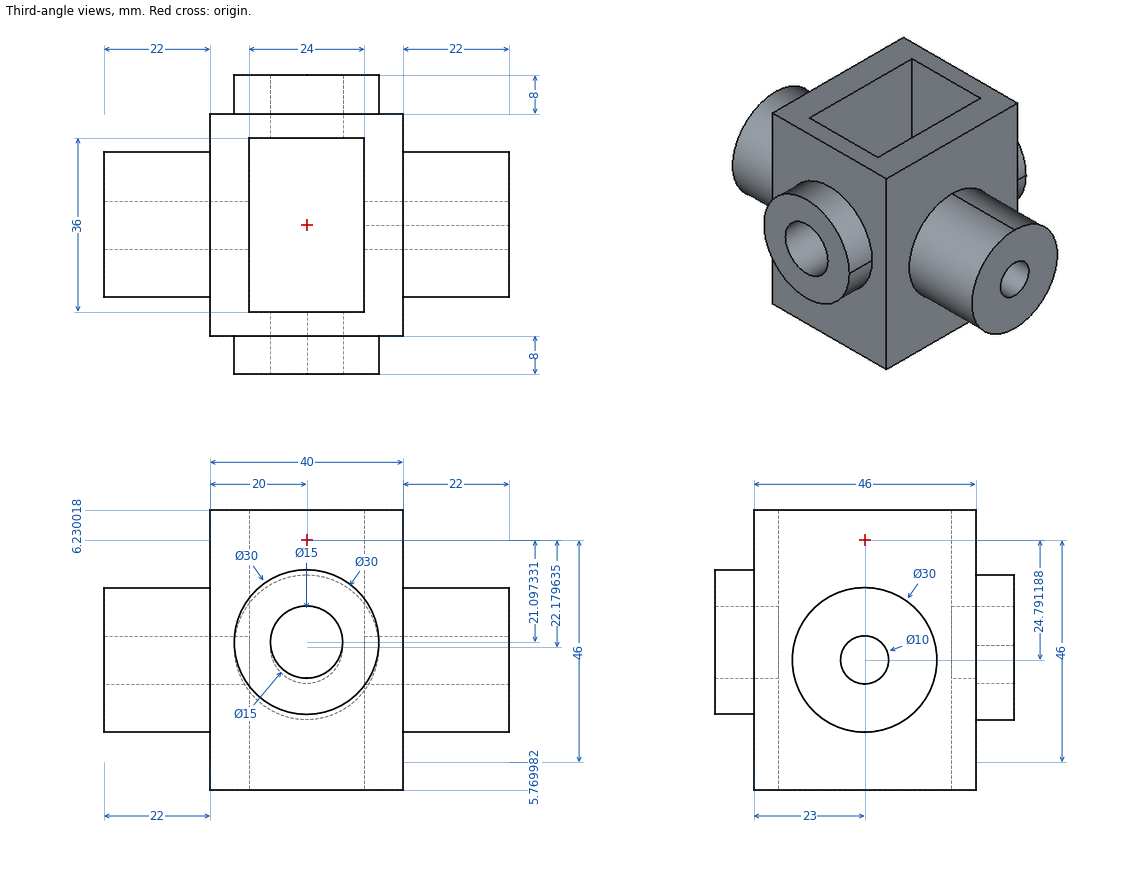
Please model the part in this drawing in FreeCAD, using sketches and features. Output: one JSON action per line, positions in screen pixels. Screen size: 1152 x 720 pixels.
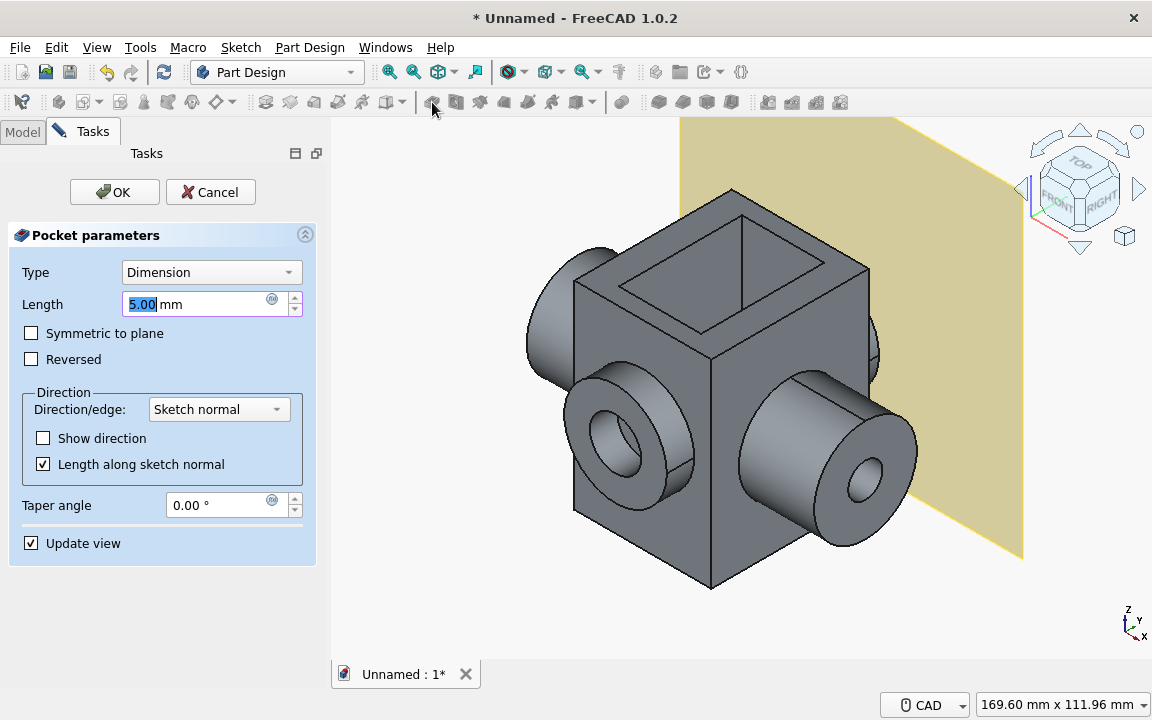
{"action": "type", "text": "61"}
{"action": "key", "text": "Tab"}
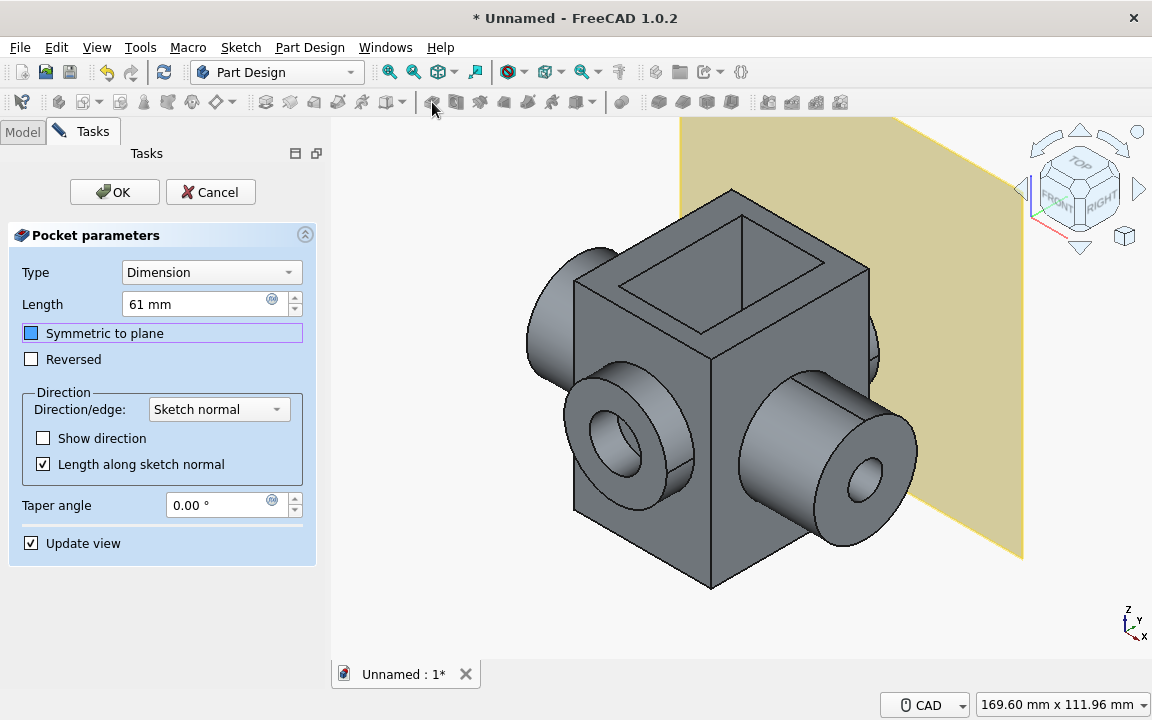
{"action": "left_click", "coordinate": [30, 359]}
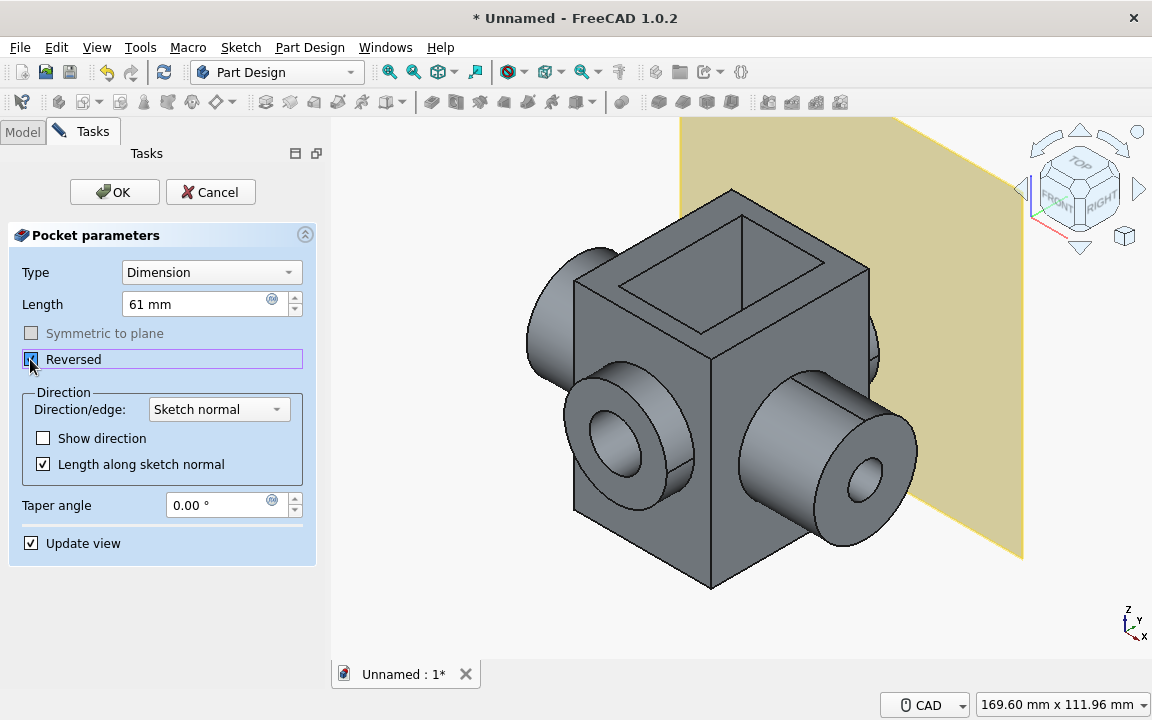
{"action": "left_click", "coordinate": [115, 192]}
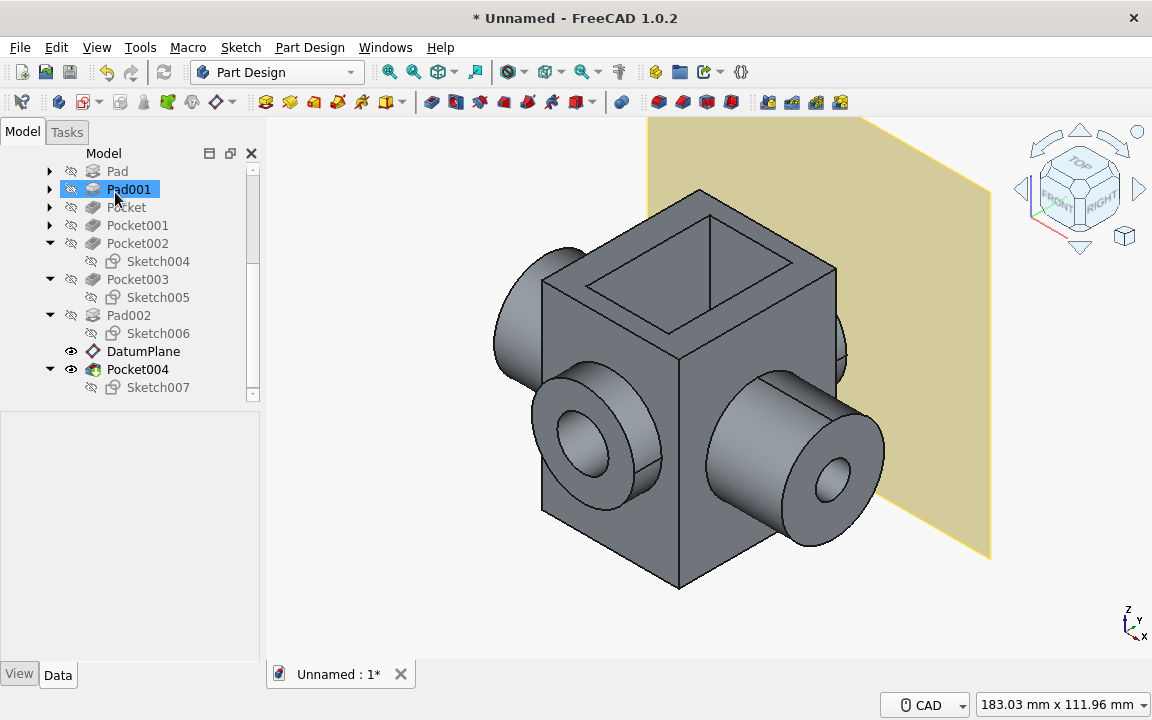
{"action": "left_click", "coordinate": [116, 351]}
{"action": "key", "text": "space"}